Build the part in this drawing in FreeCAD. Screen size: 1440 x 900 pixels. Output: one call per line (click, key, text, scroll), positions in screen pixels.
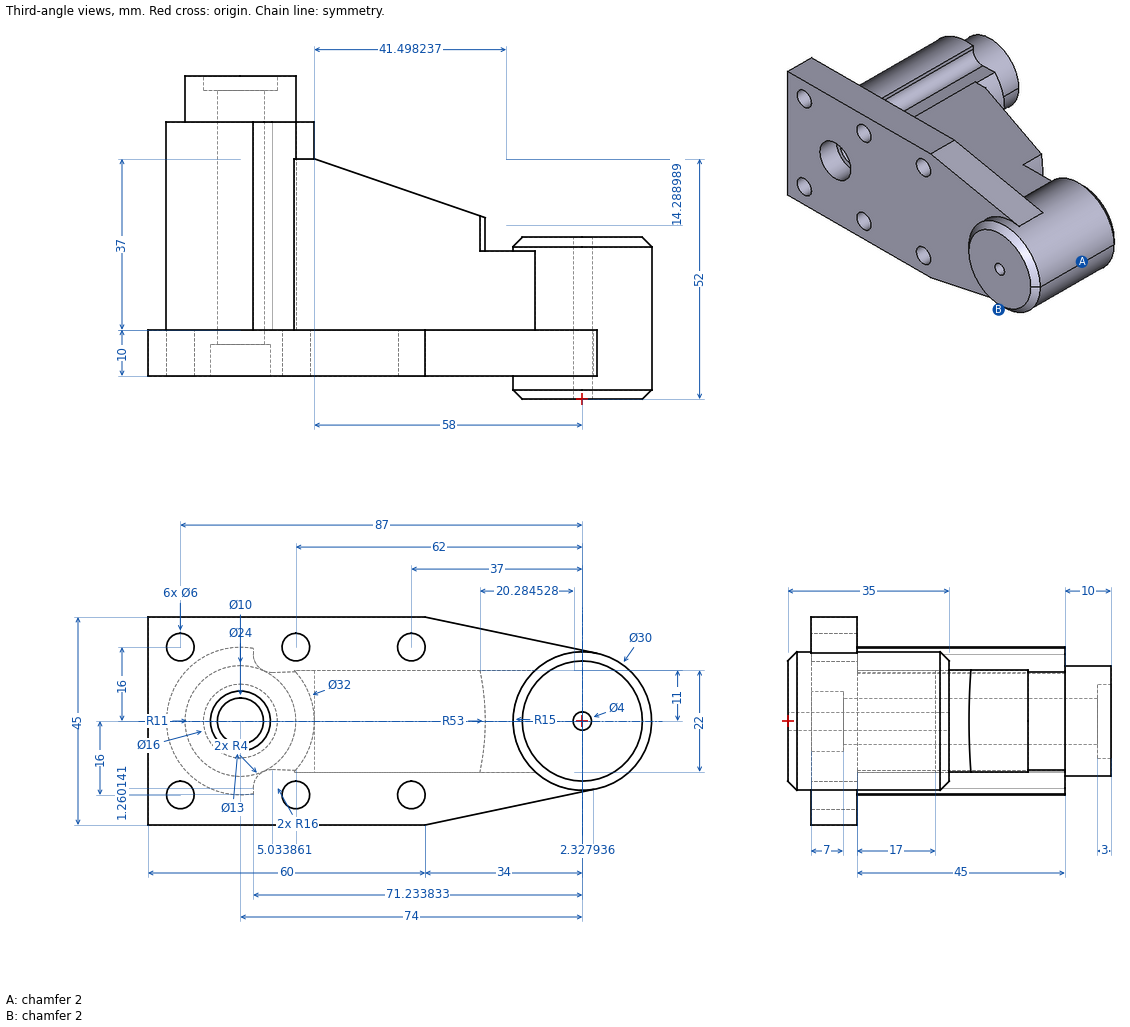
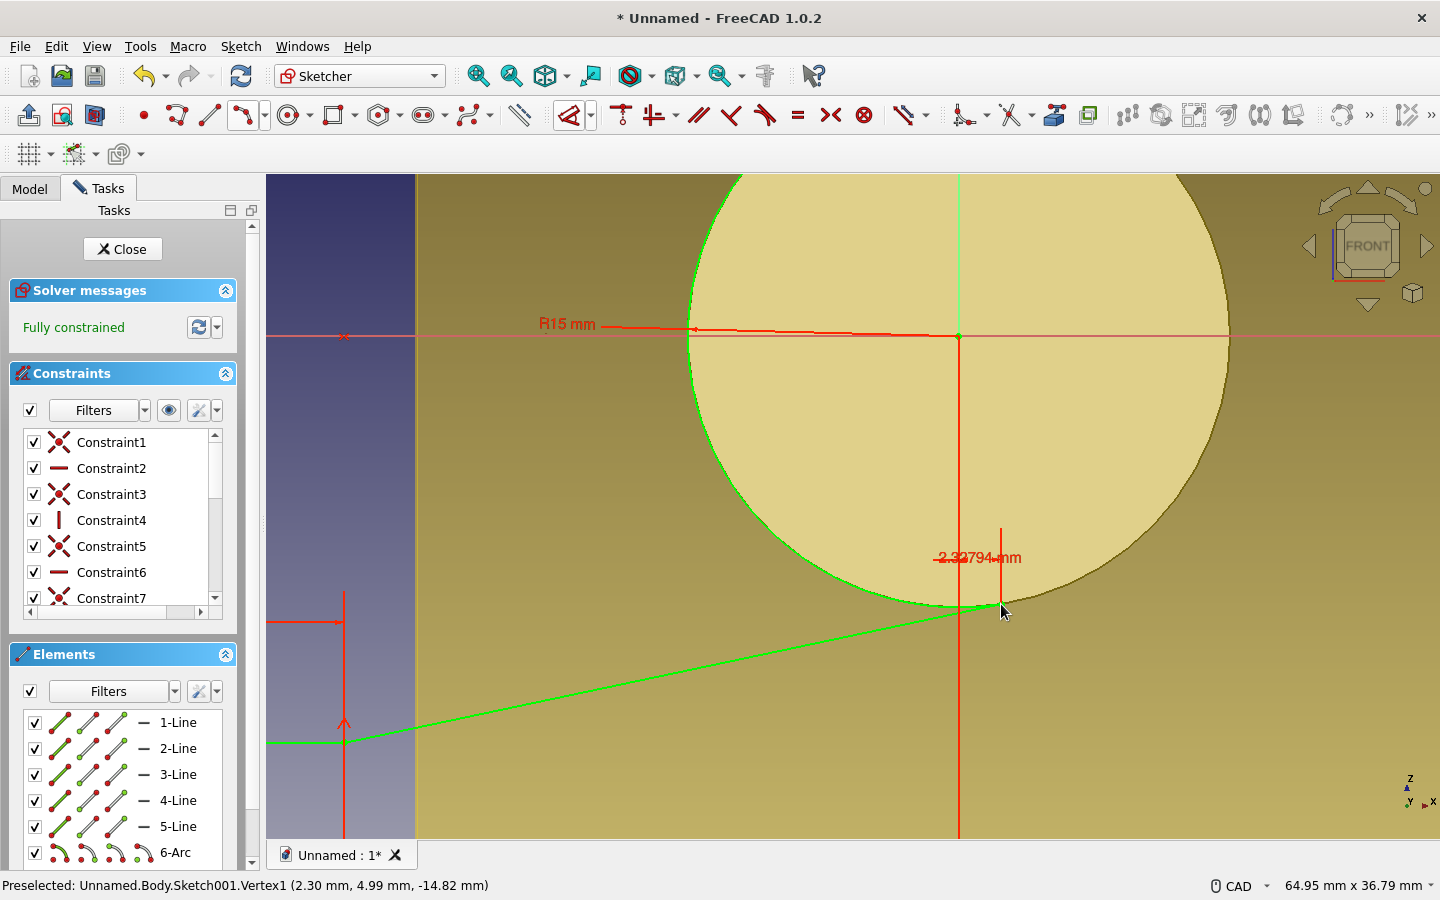
click(123, 249)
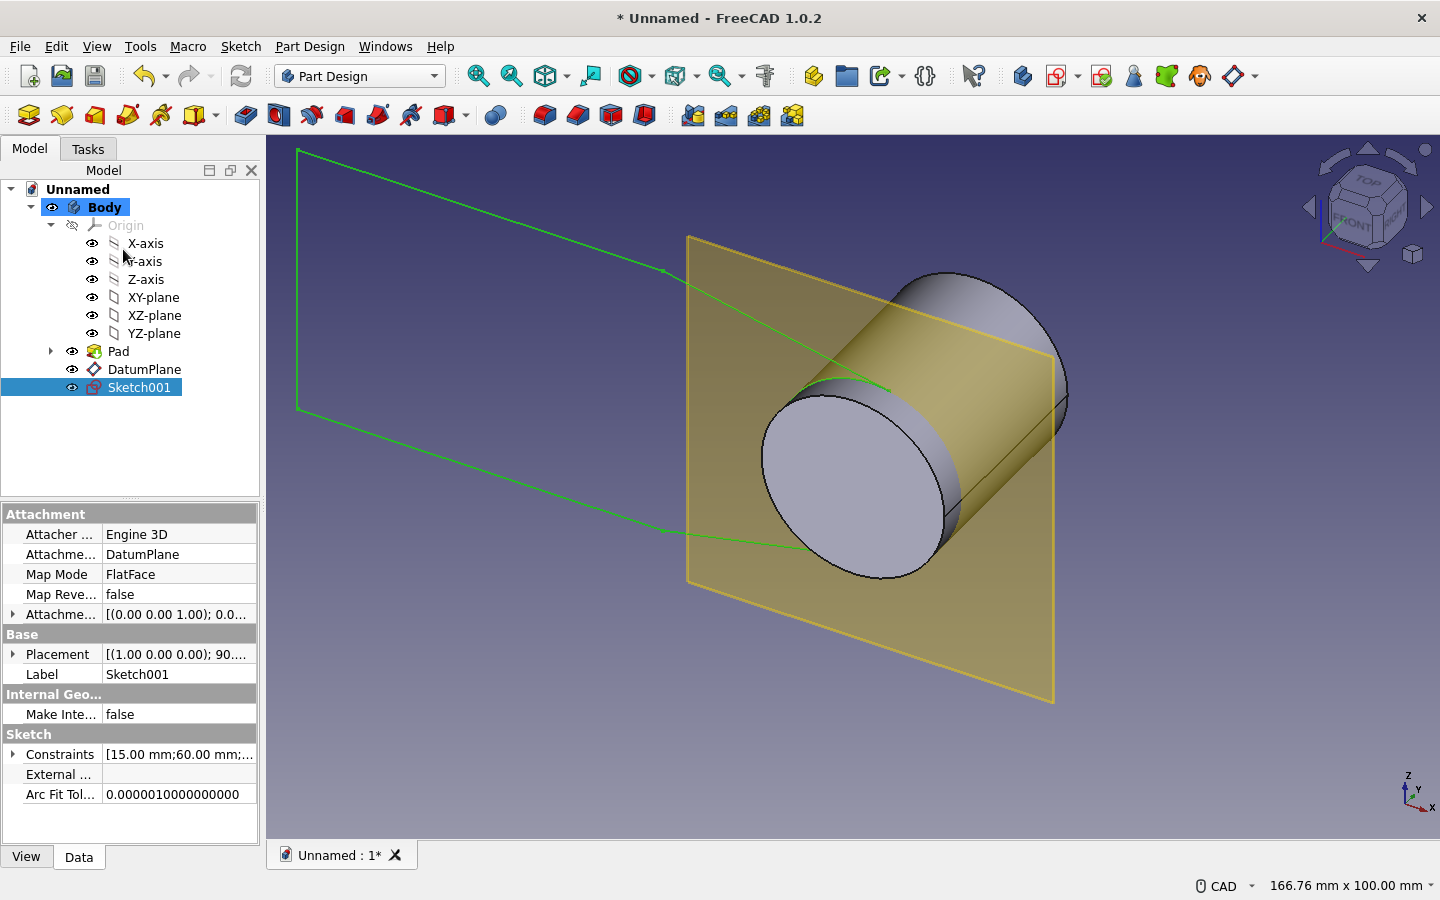
click(29, 116)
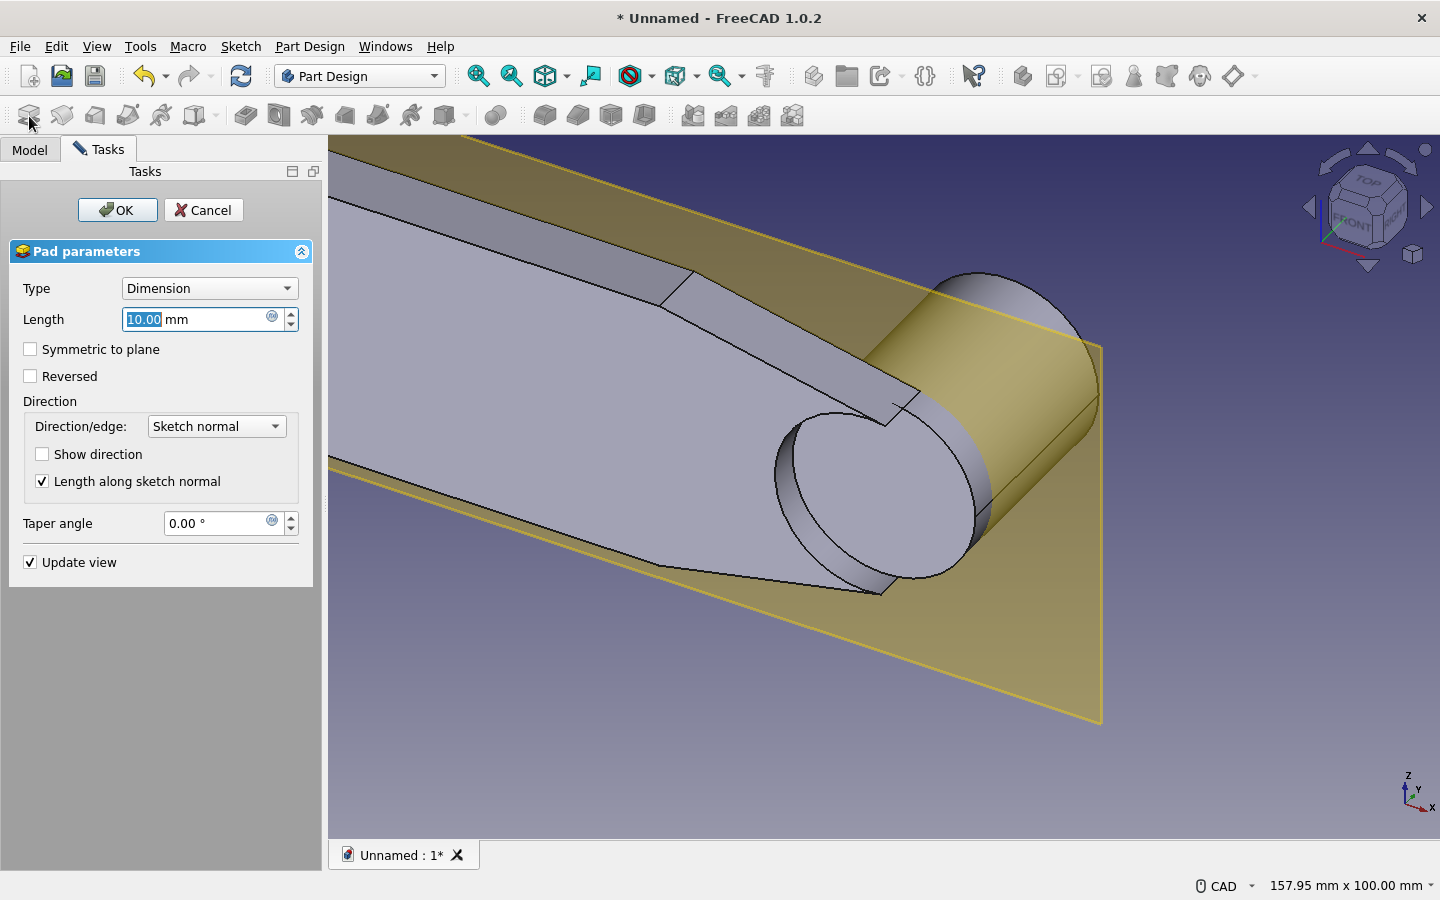
text(10)
key(Tab)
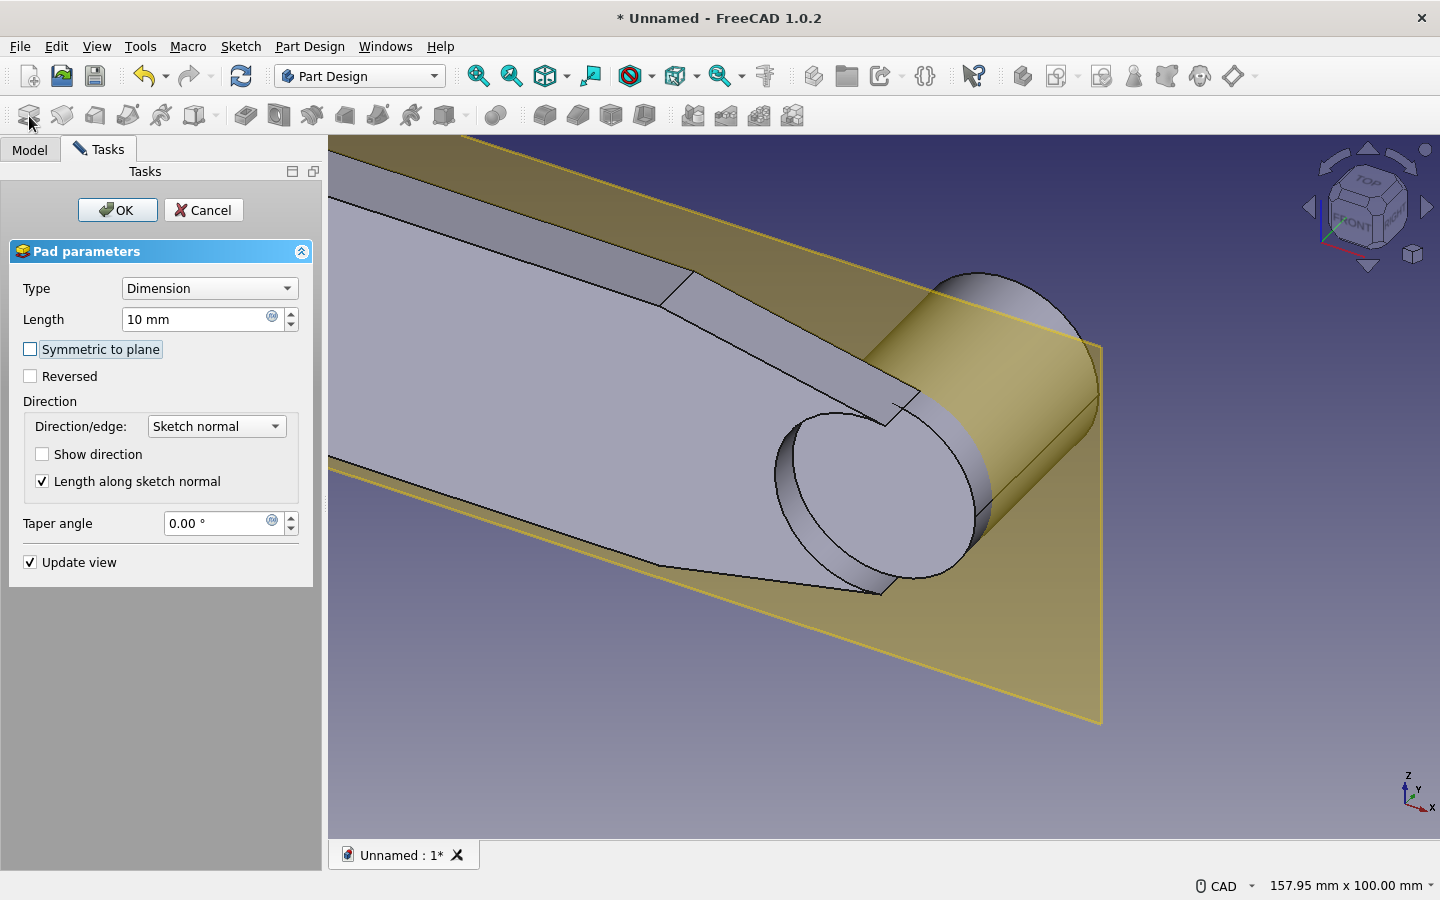
click(31, 376)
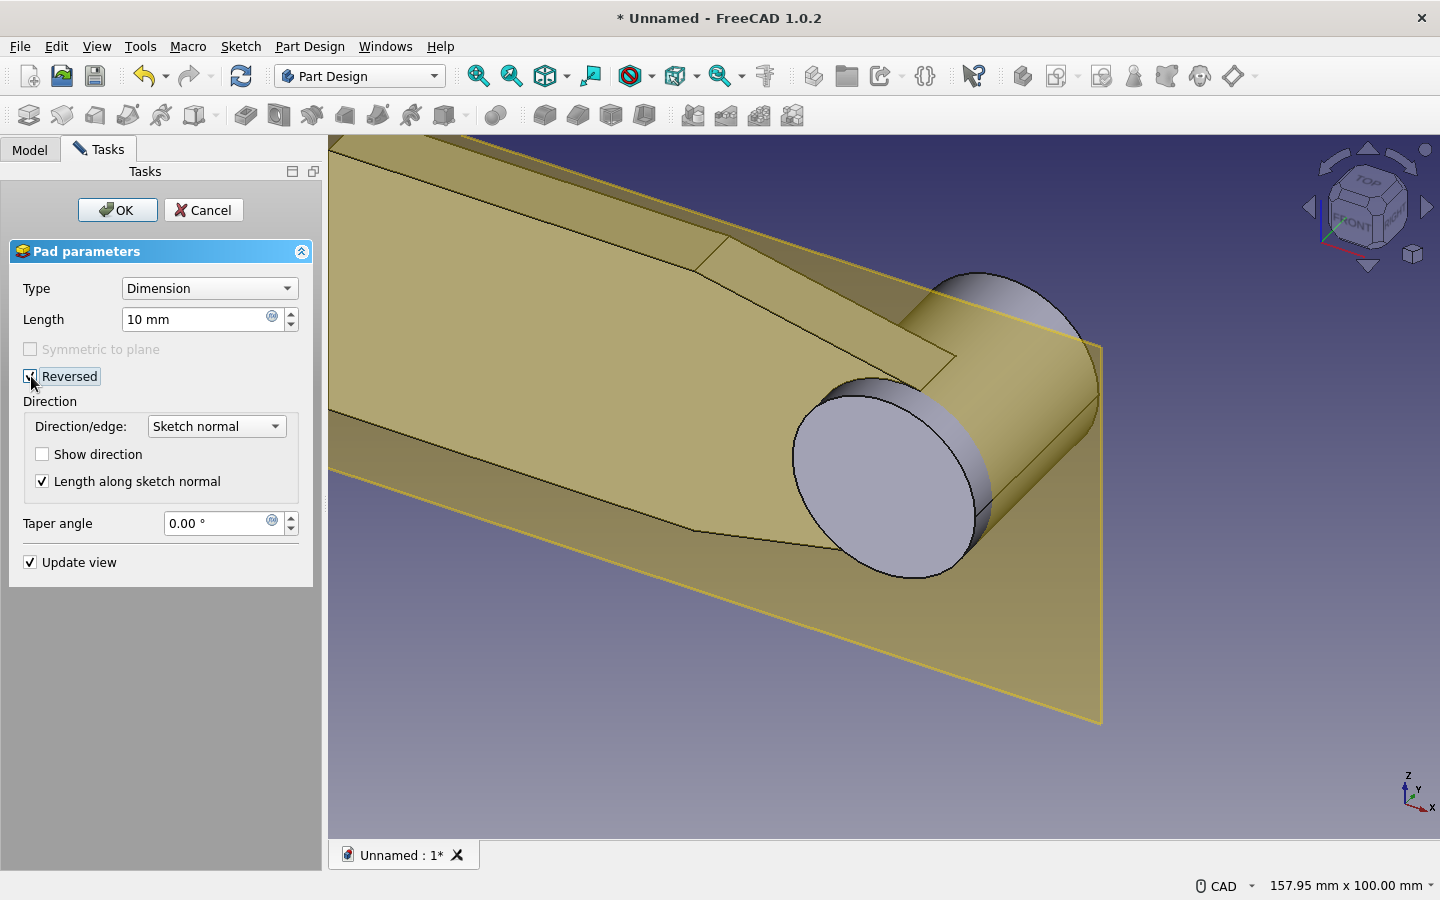
click(118, 210)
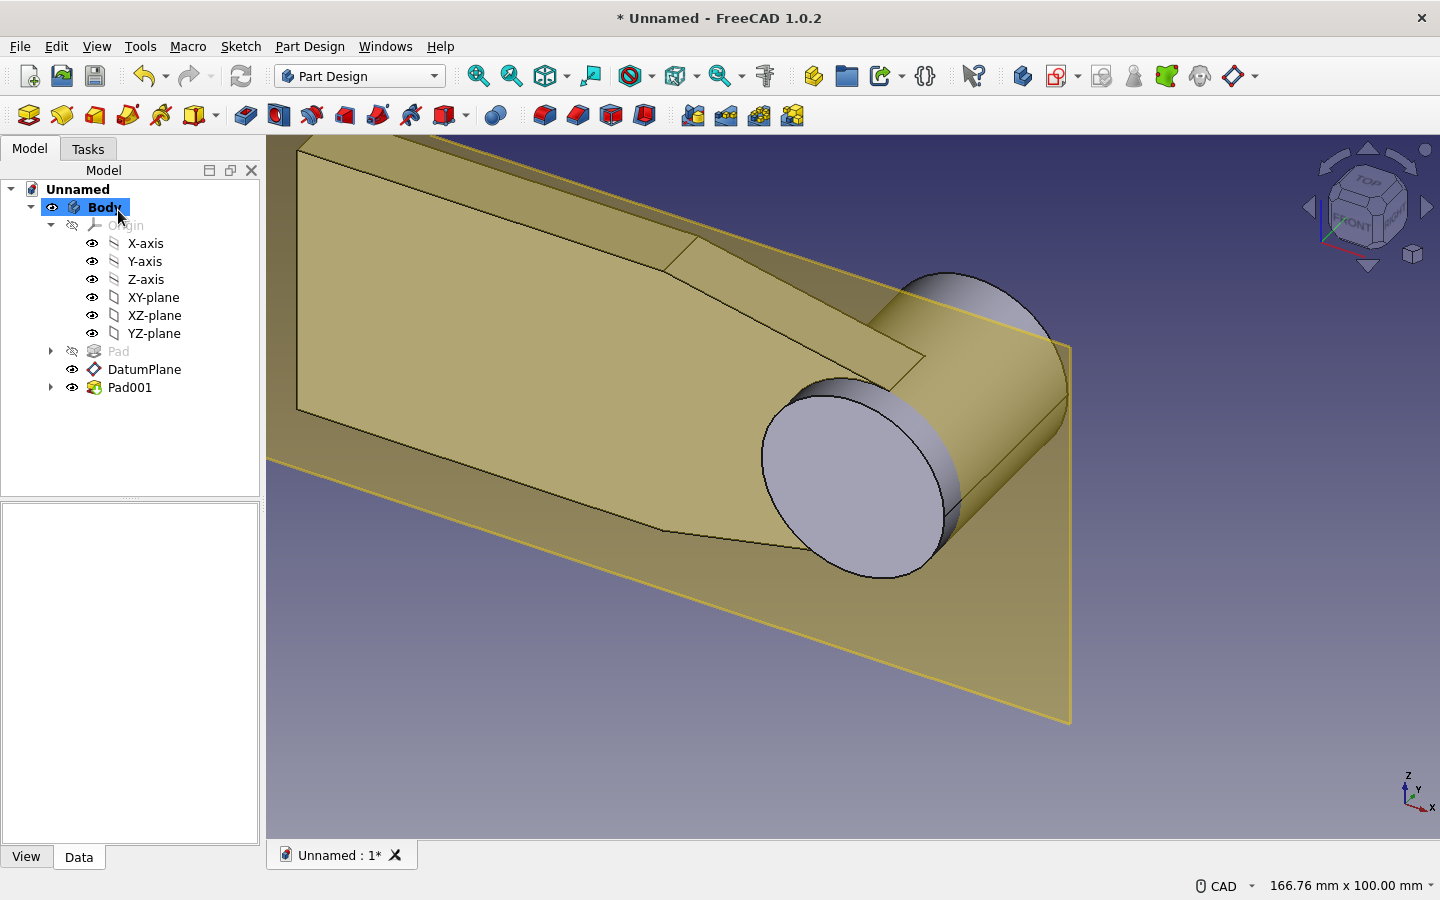
click(117, 369)
key(space)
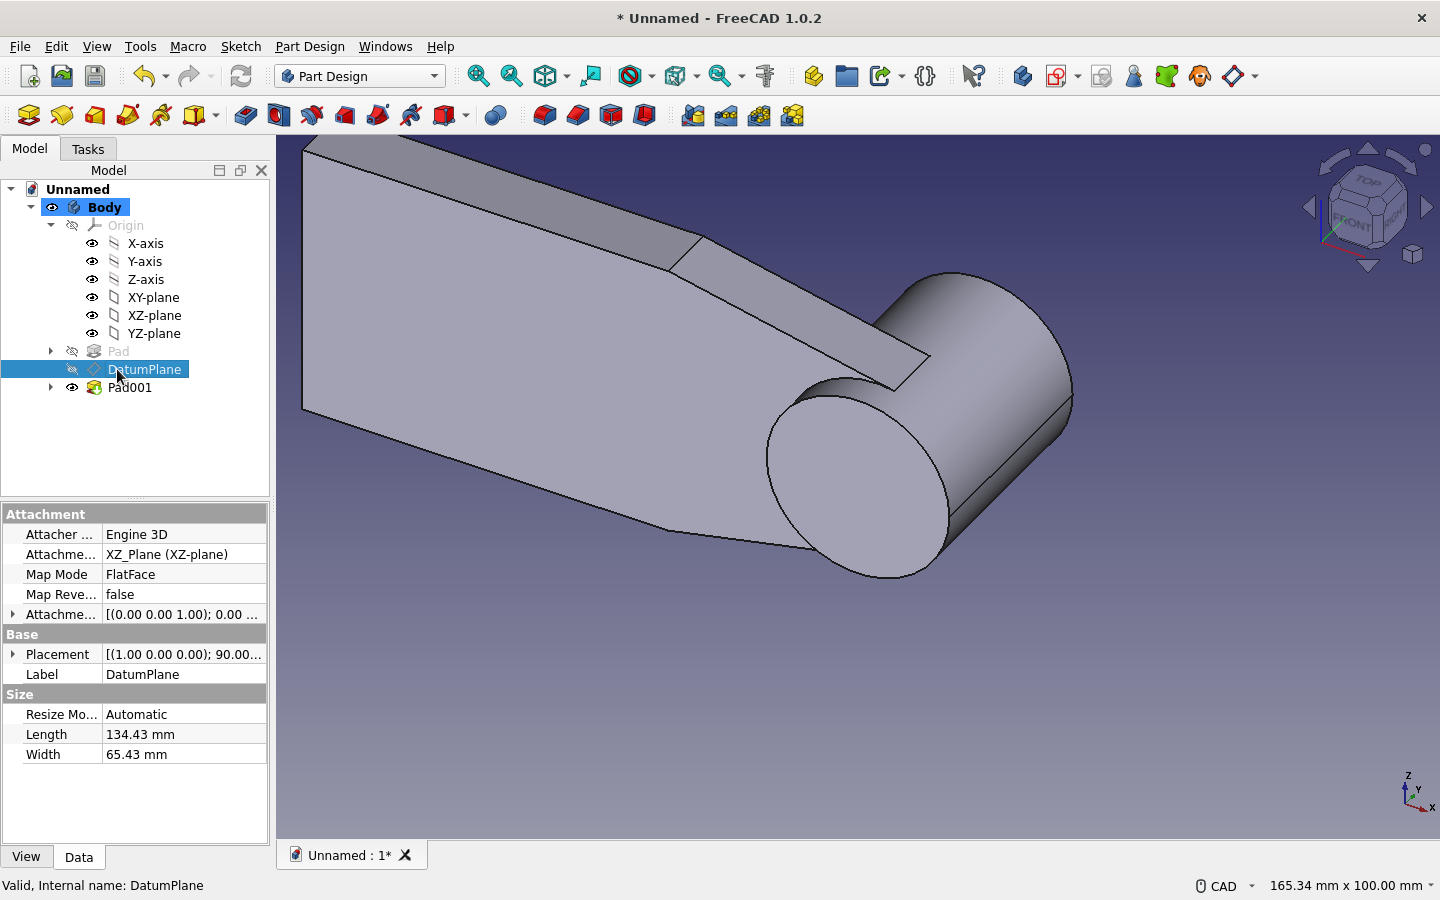
click(479, 76)